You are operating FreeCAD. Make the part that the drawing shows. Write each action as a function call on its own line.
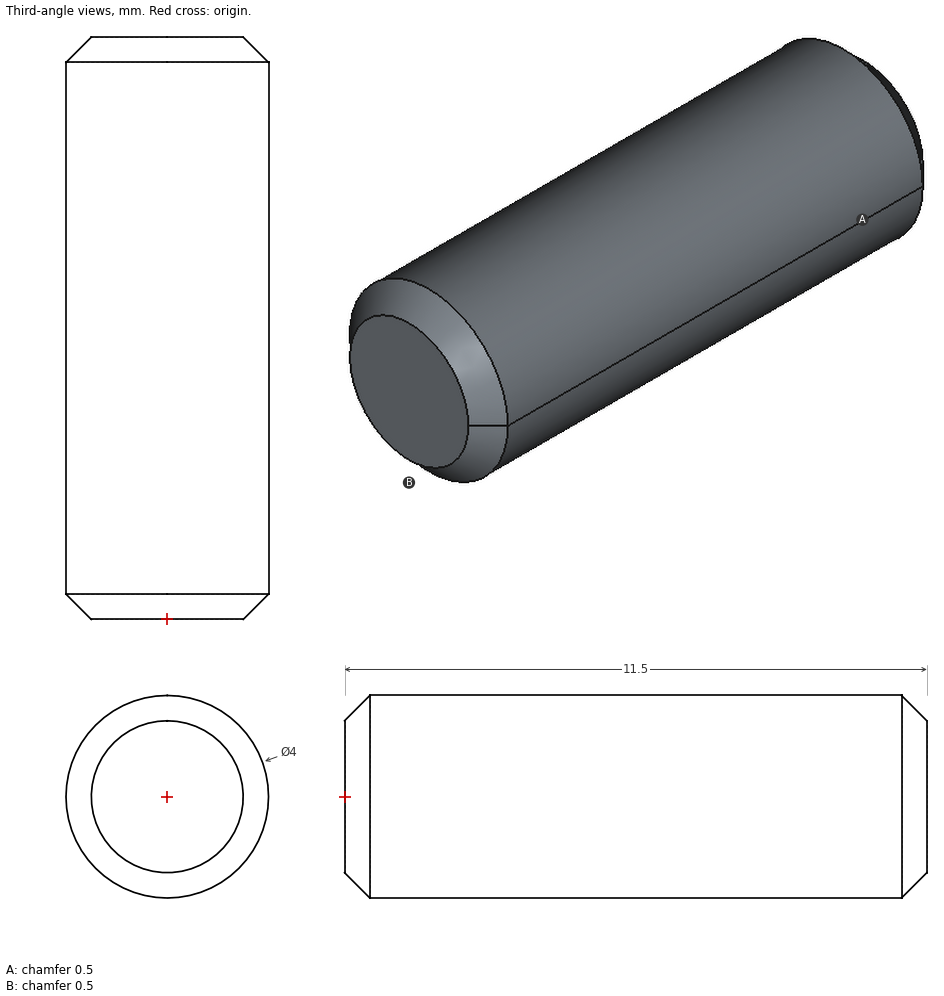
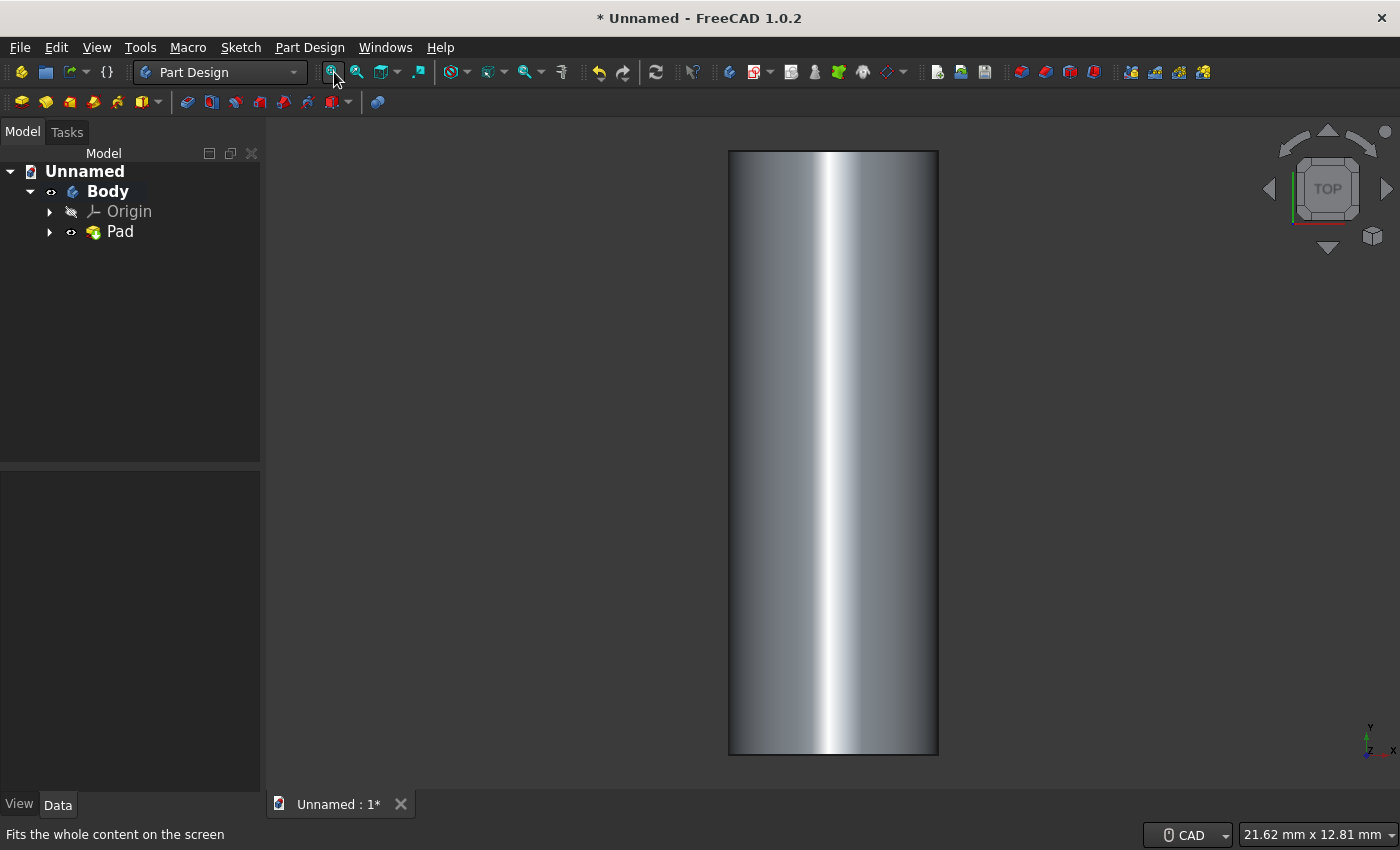
click(748, 150)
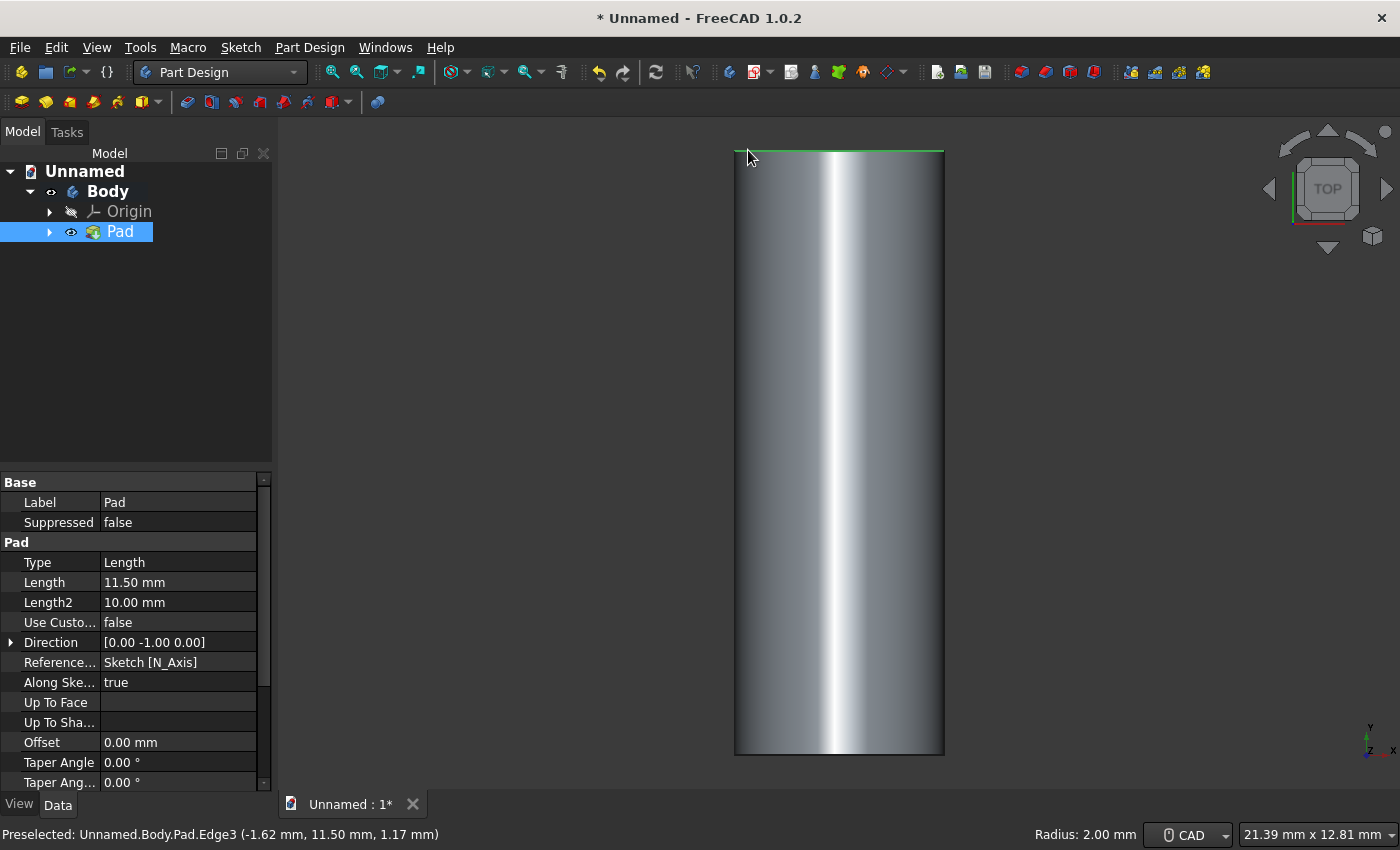
click(1046, 72)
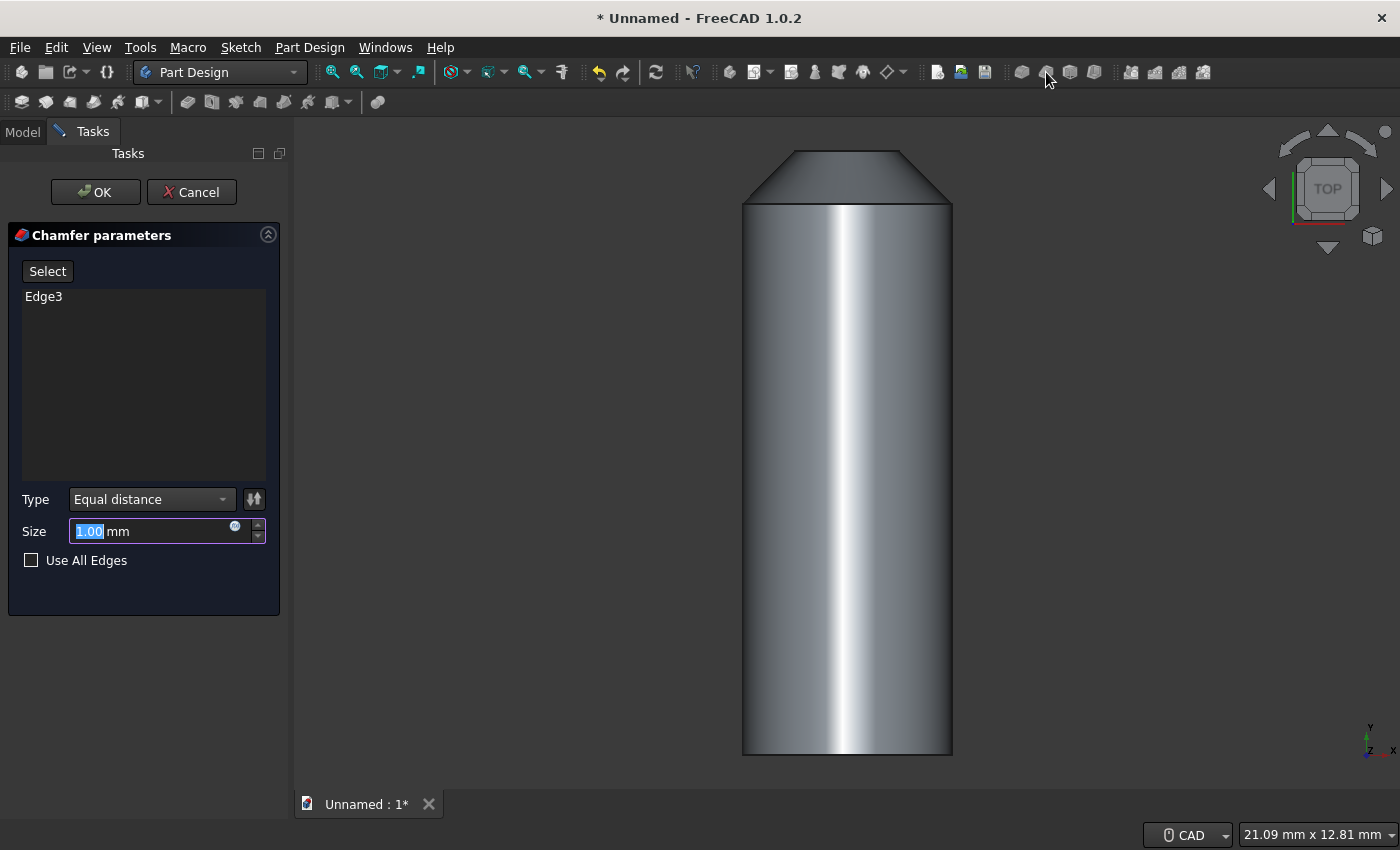
text(0.5)
key(Tab)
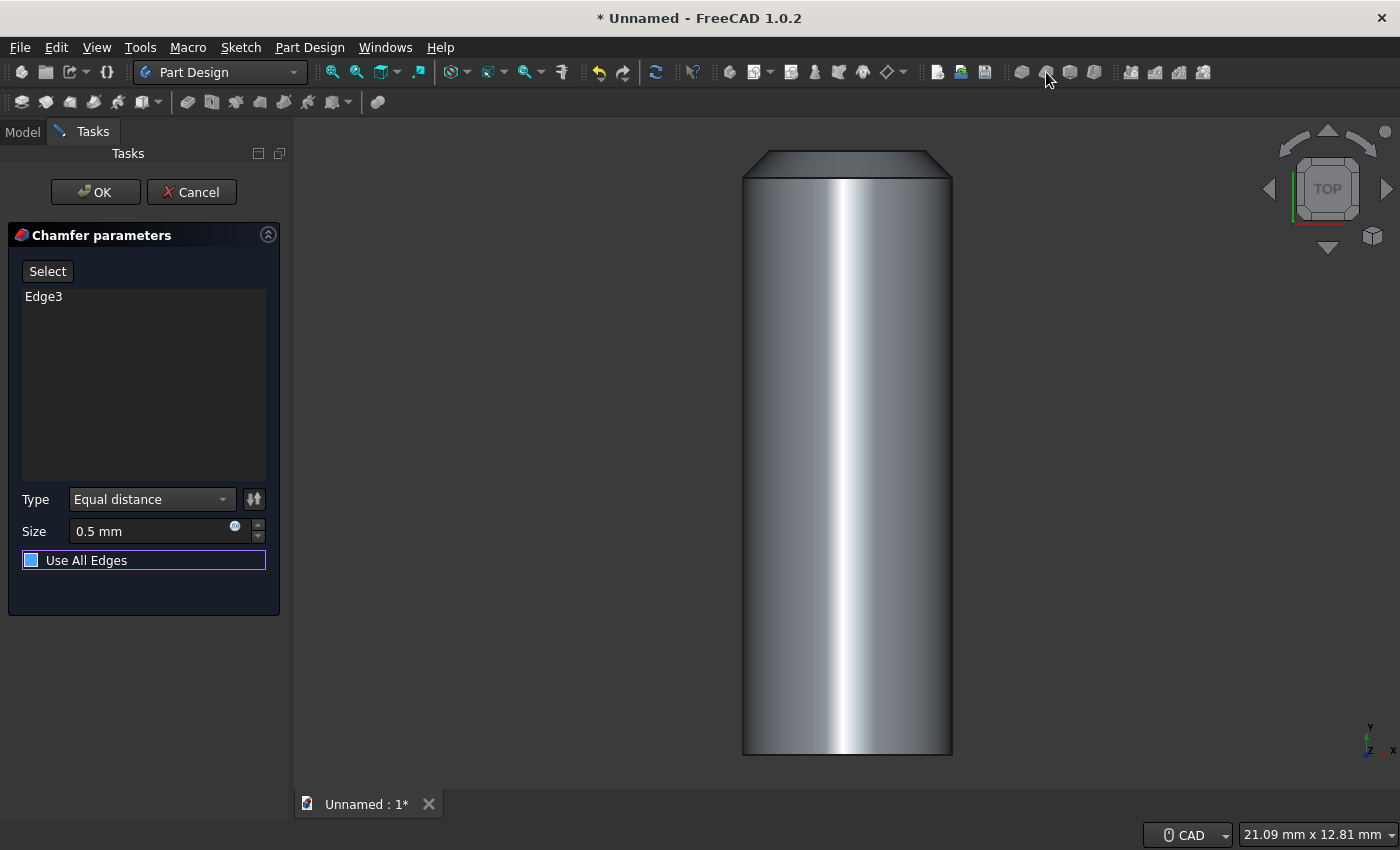
click(96, 192)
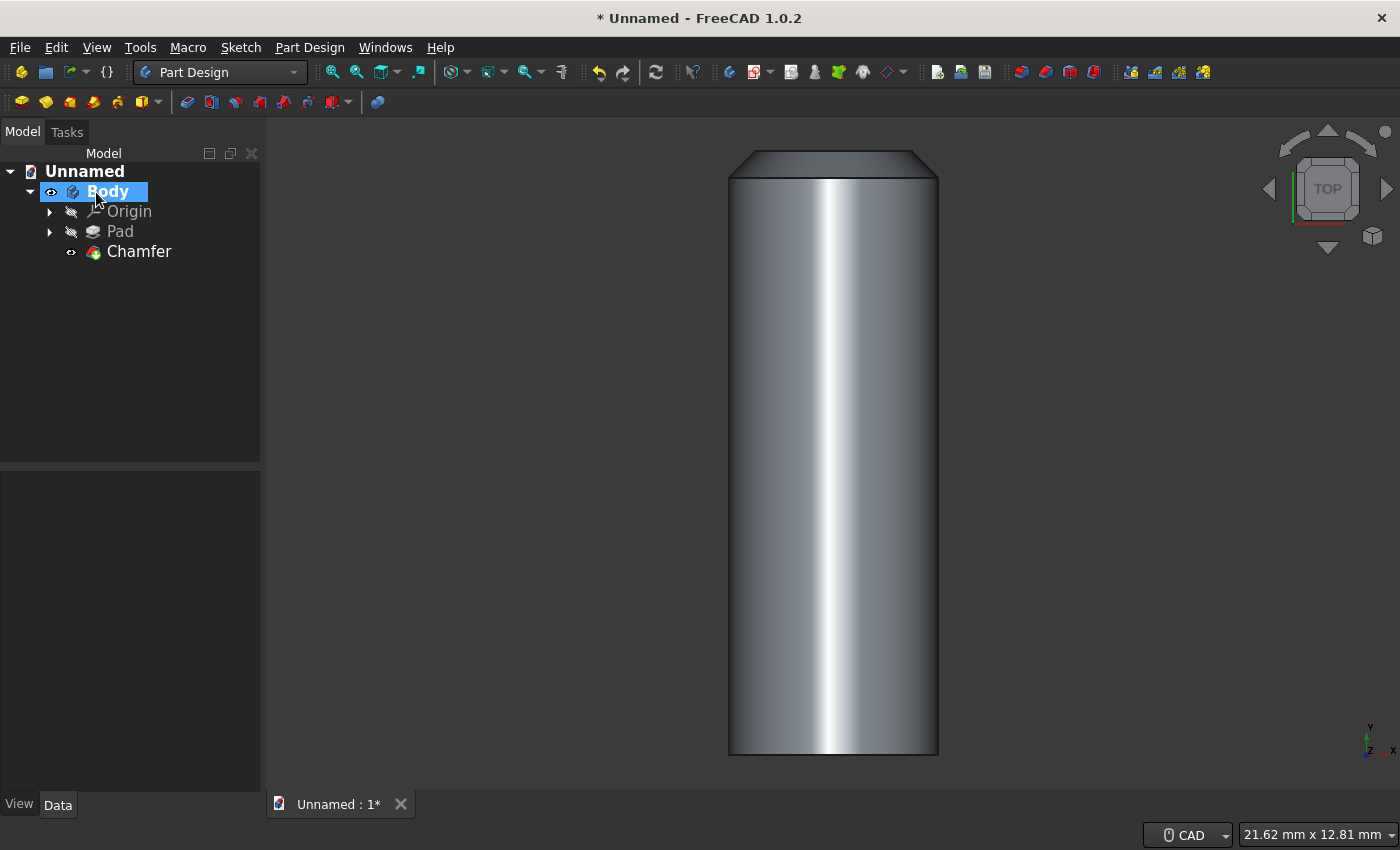
click(865, 754)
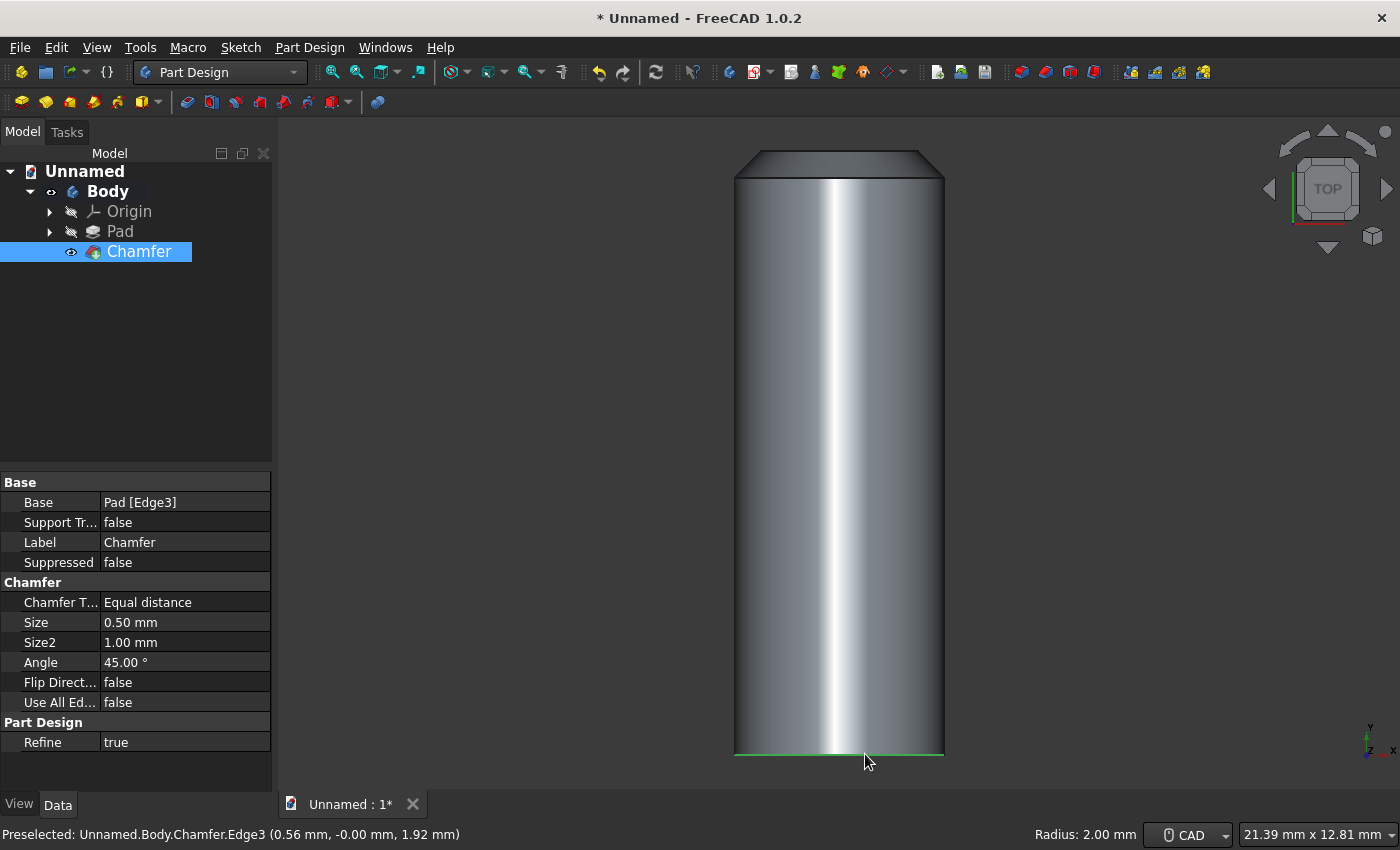
click(1046, 72)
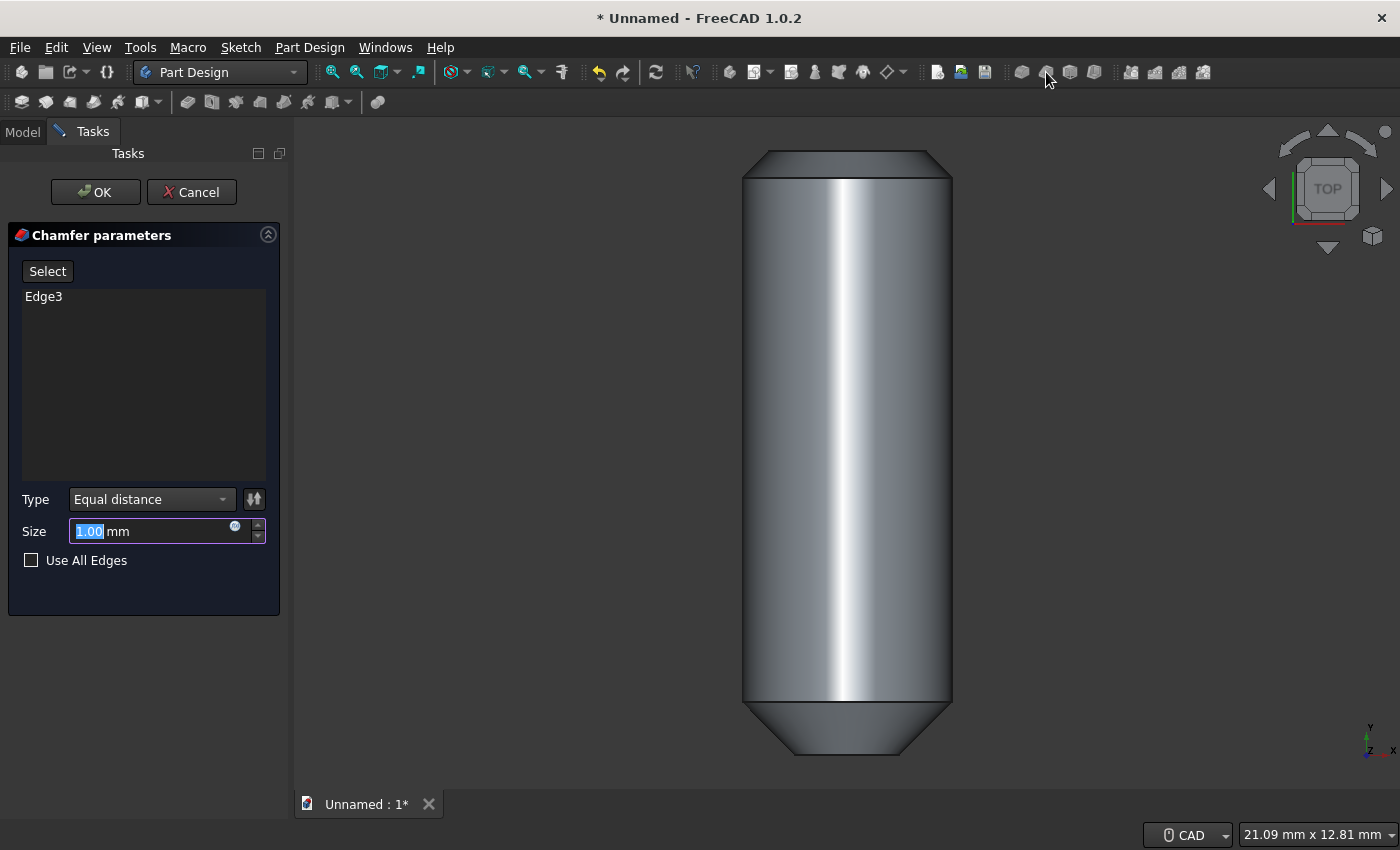
text(0.5)
key(Tab)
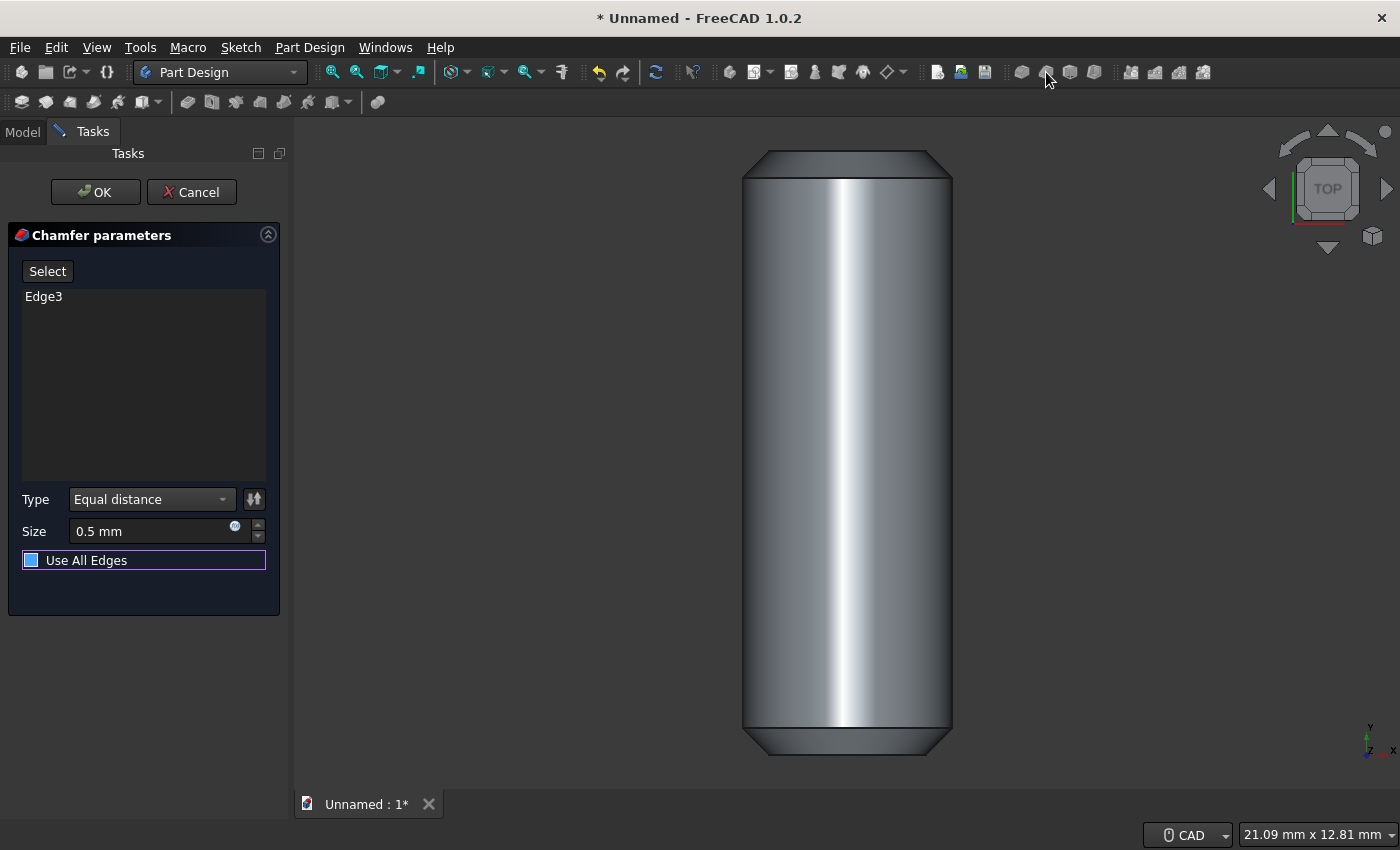
click(96, 192)